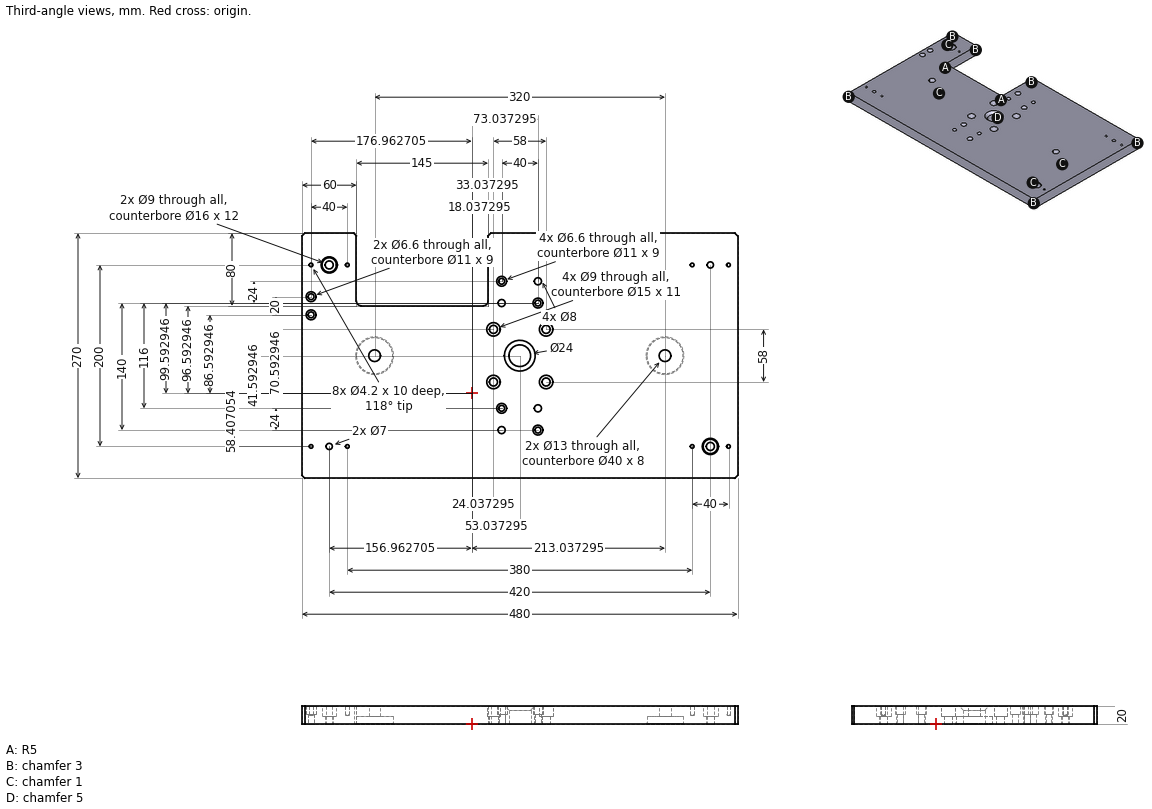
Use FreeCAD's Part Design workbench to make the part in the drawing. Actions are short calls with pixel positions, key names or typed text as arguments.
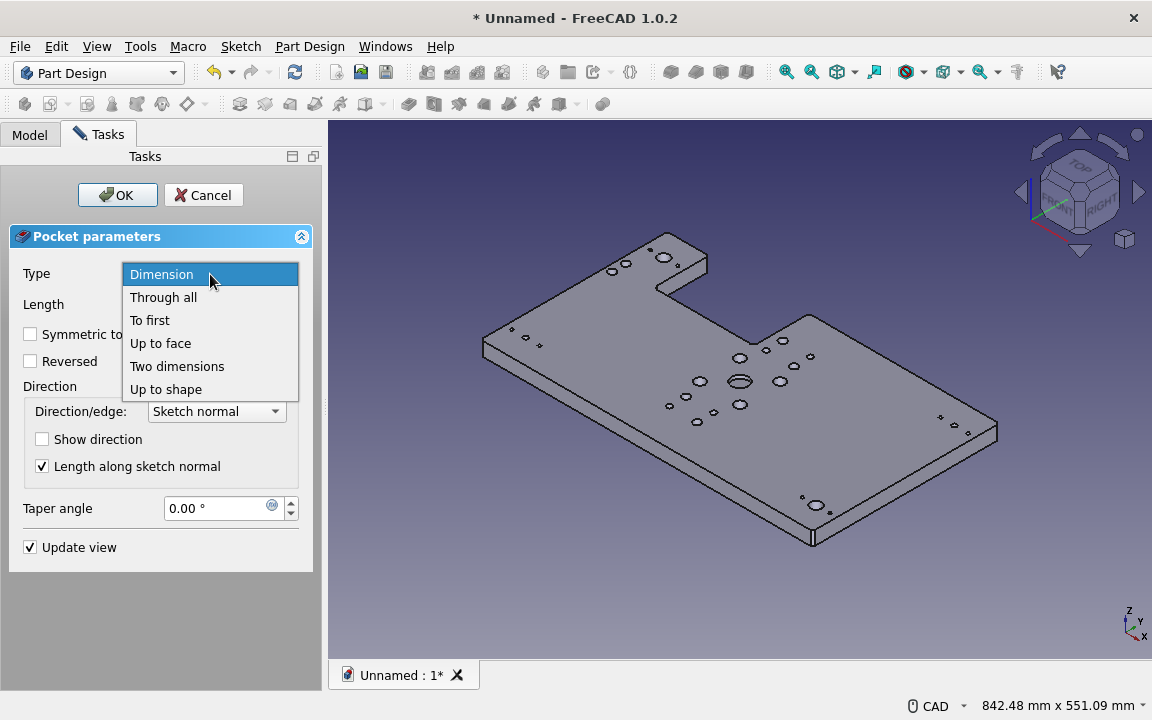
click(208, 298)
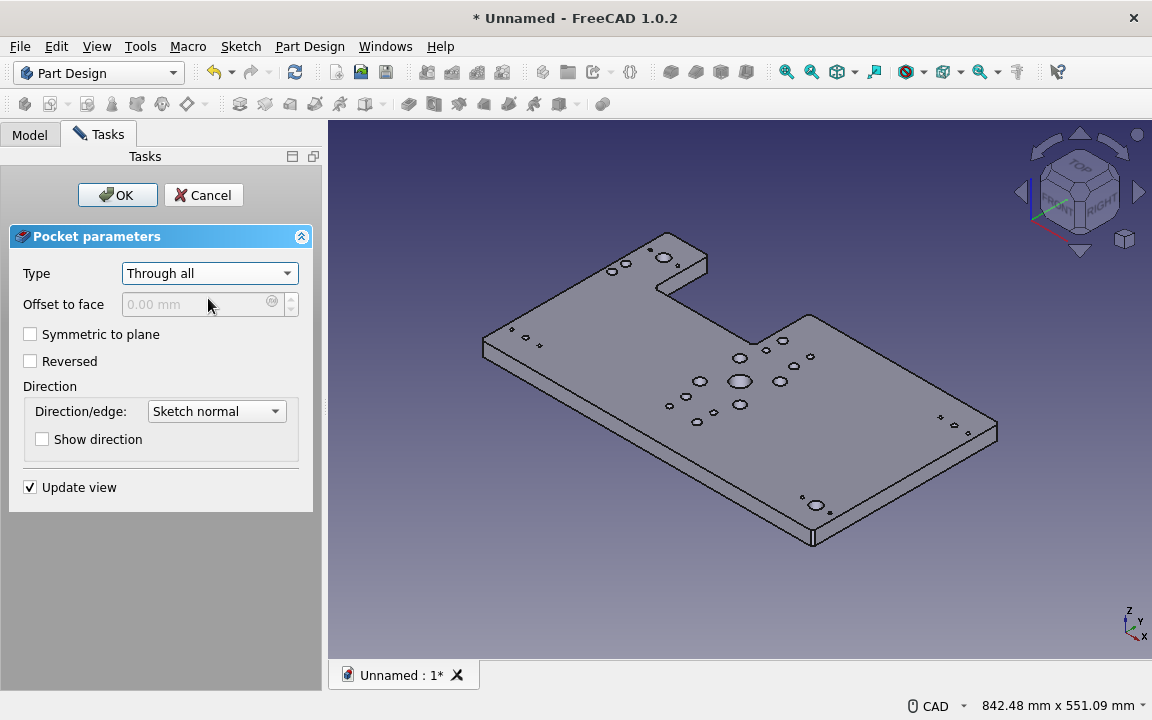
click(118, 195)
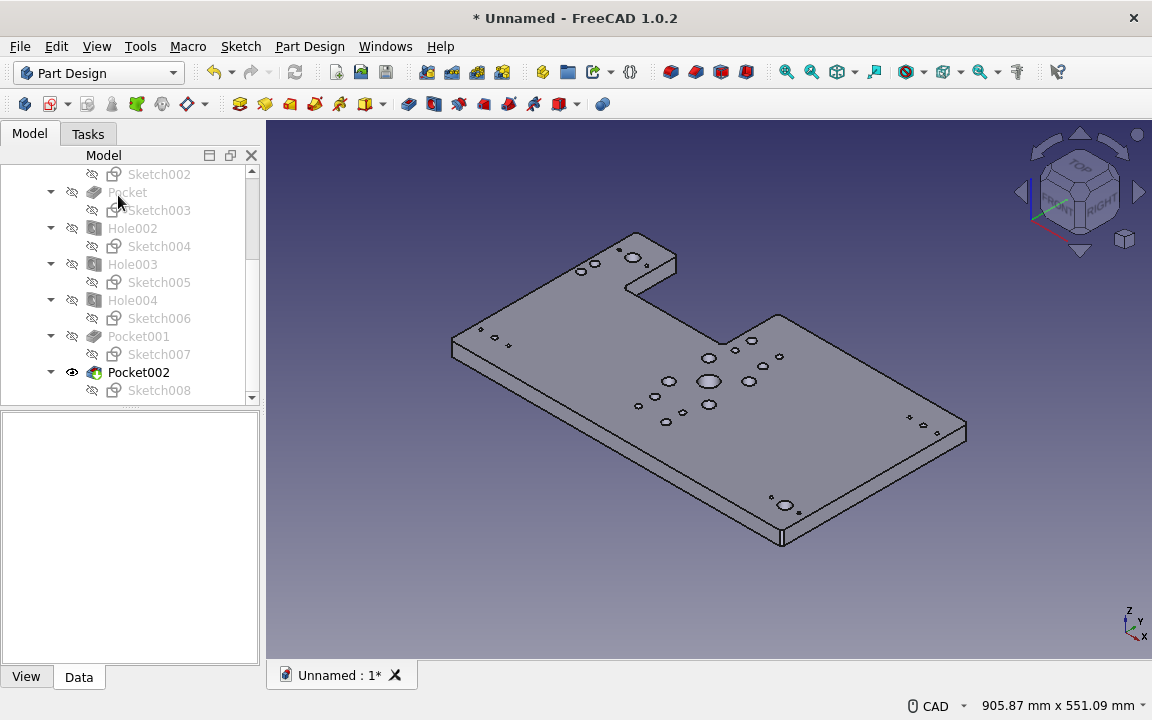
click(50, 104)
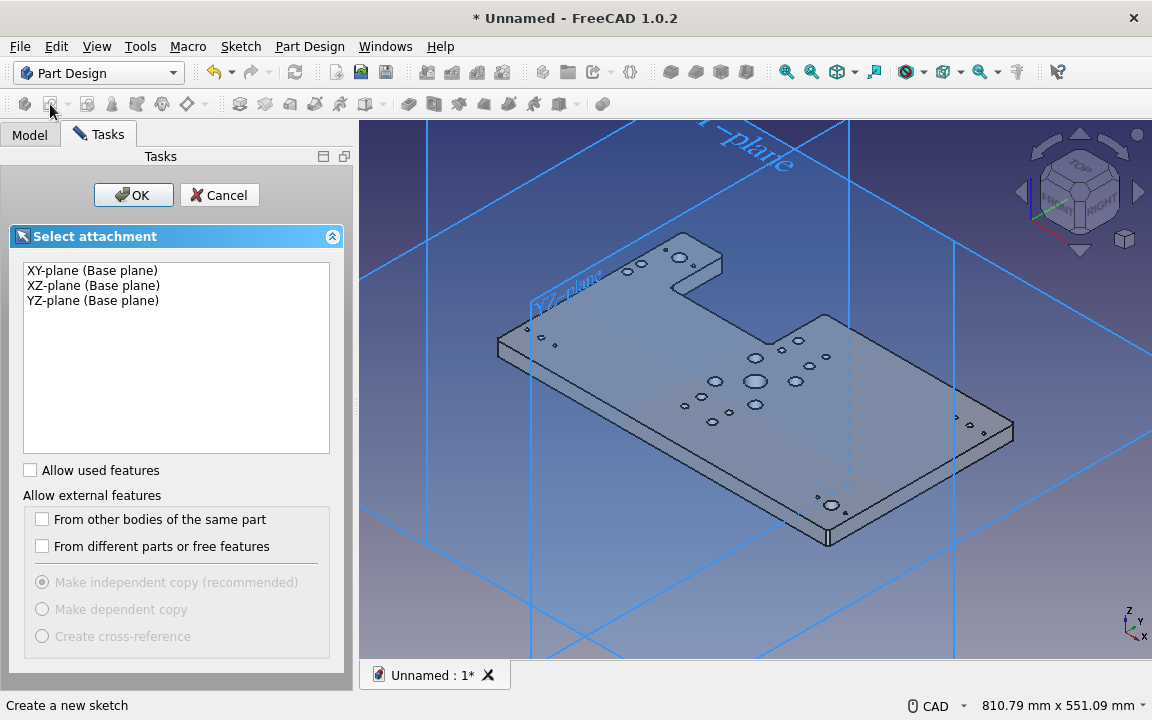
click(84, 270)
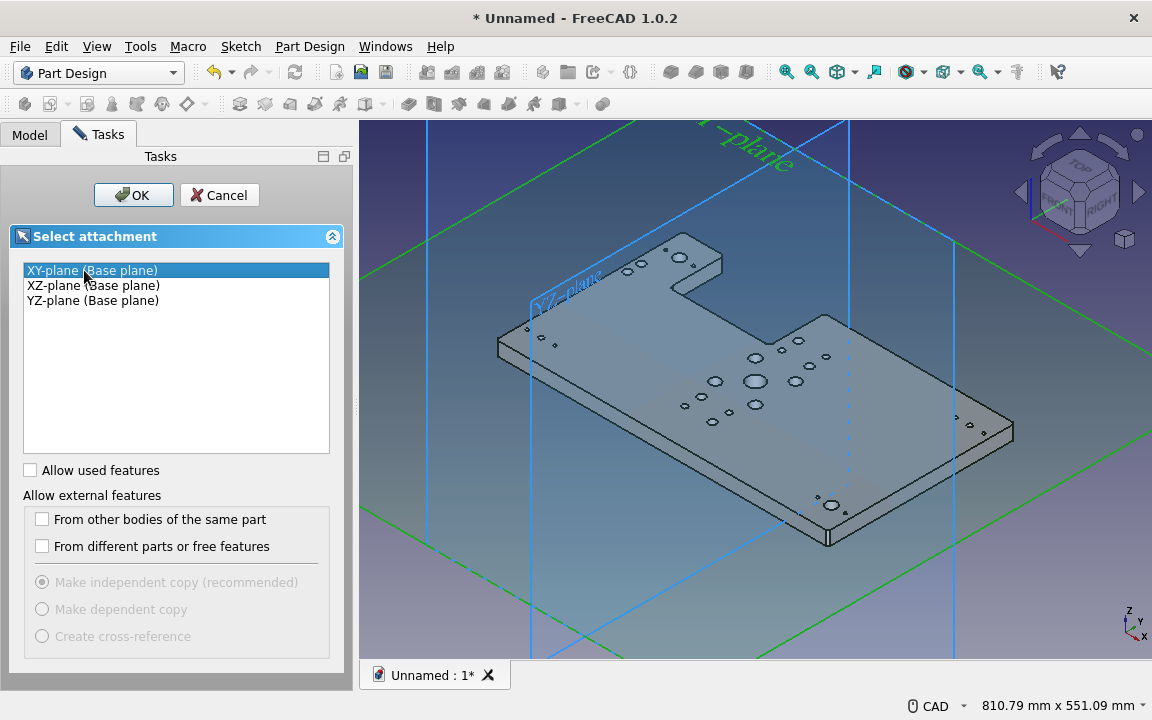
click(134, 195)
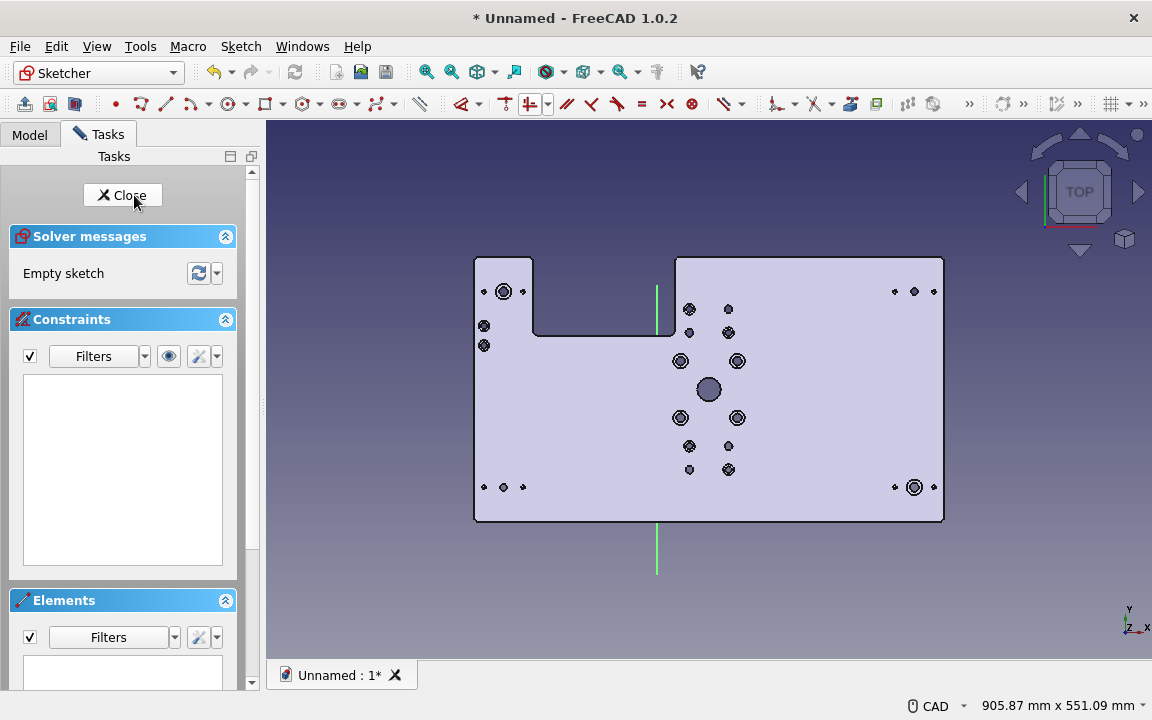
key(q)
key(s)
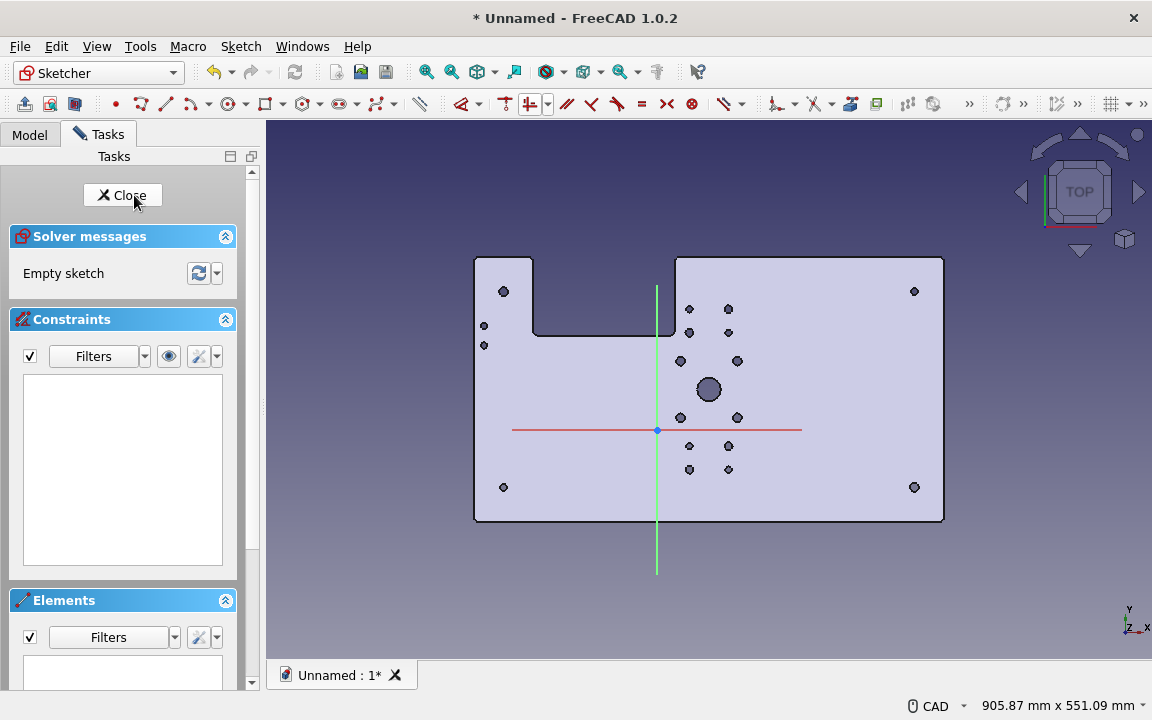
scroll(848, 442, up, 2)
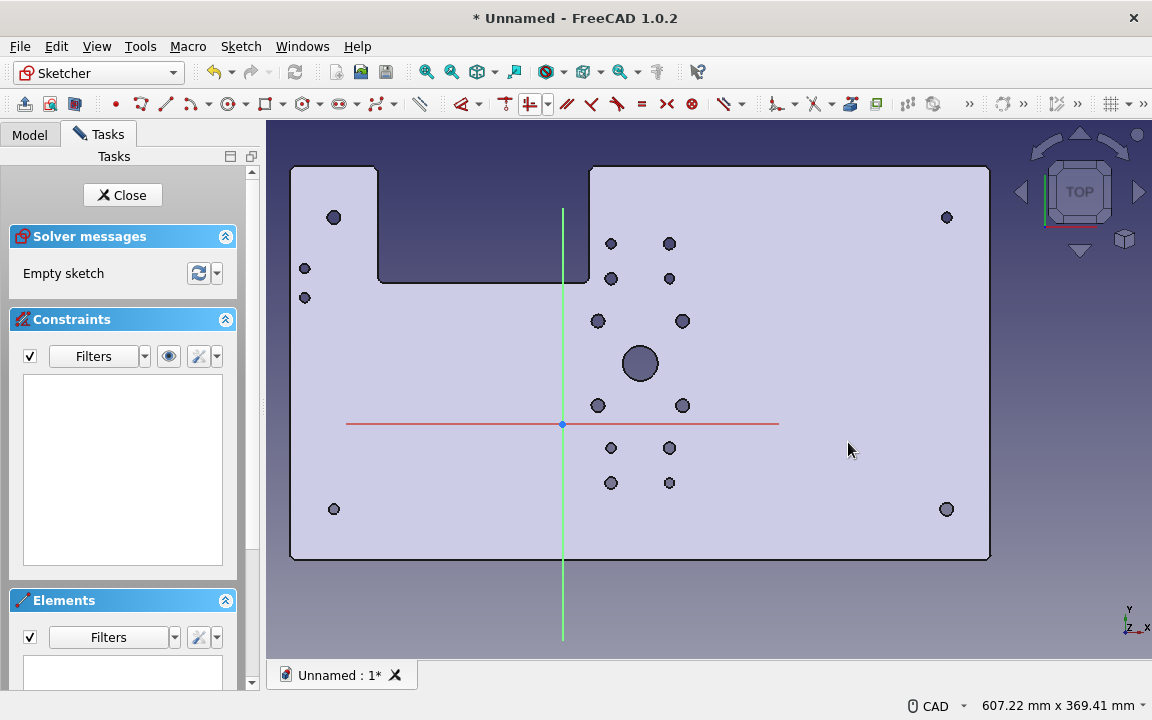
key(g)
key(c)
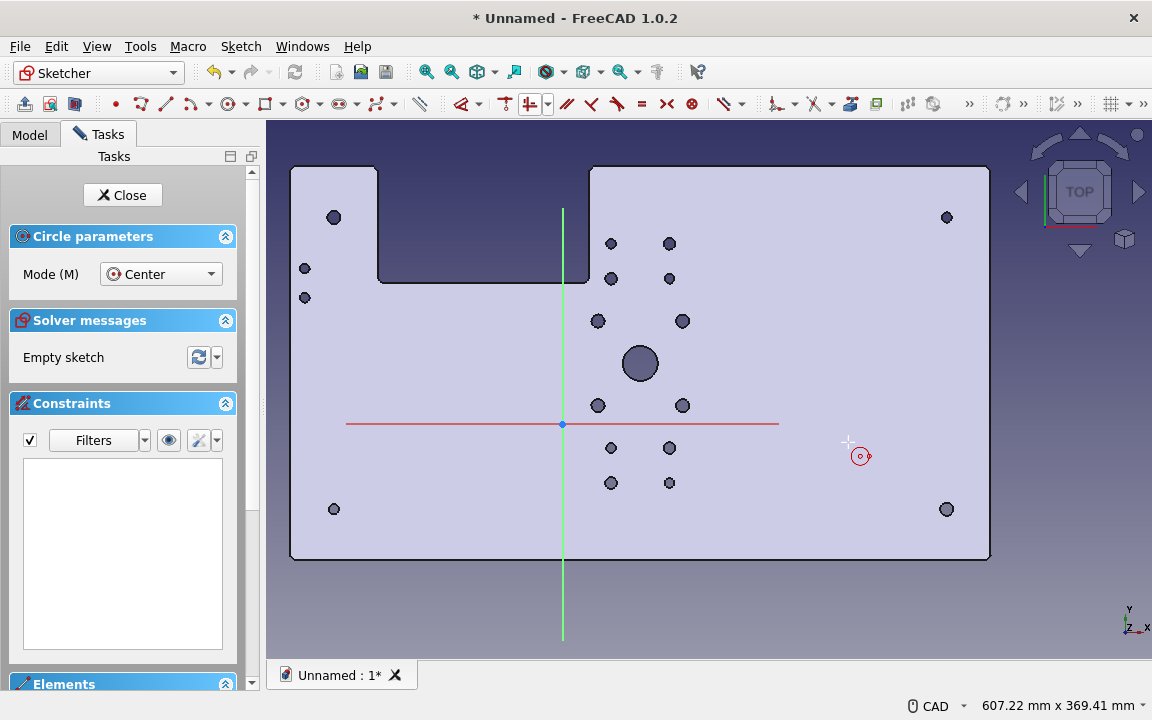
scroll(874, 363, up, 5)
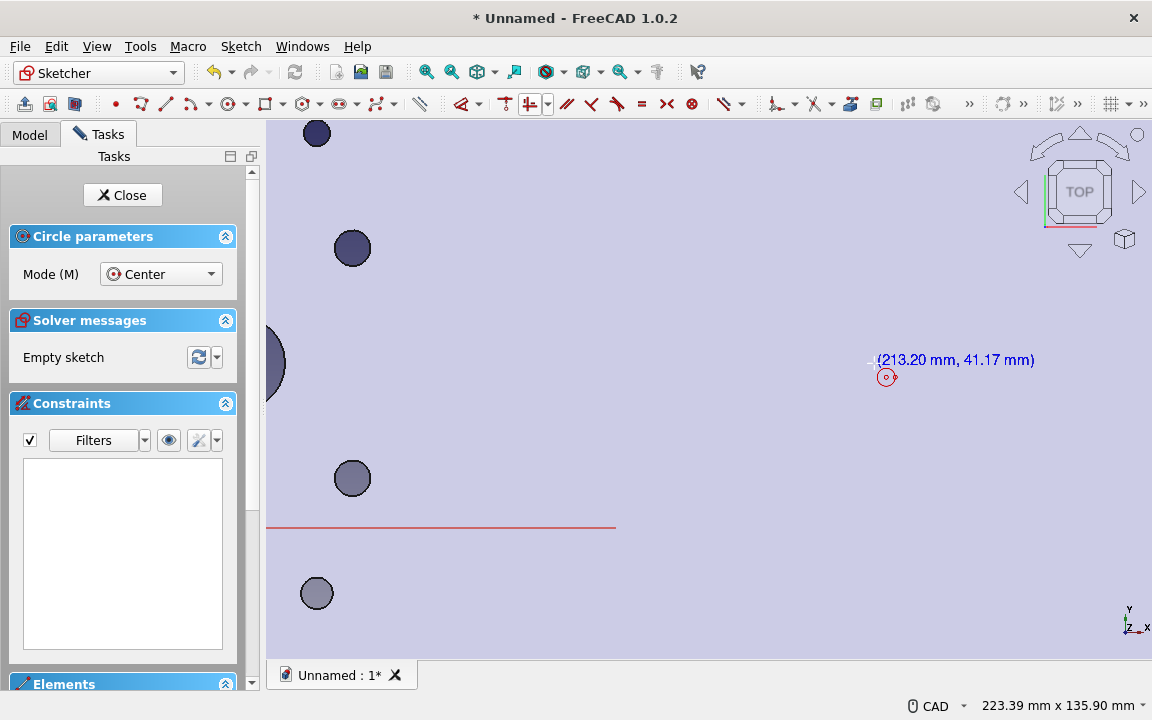
click(872, 363)
click(890, 345)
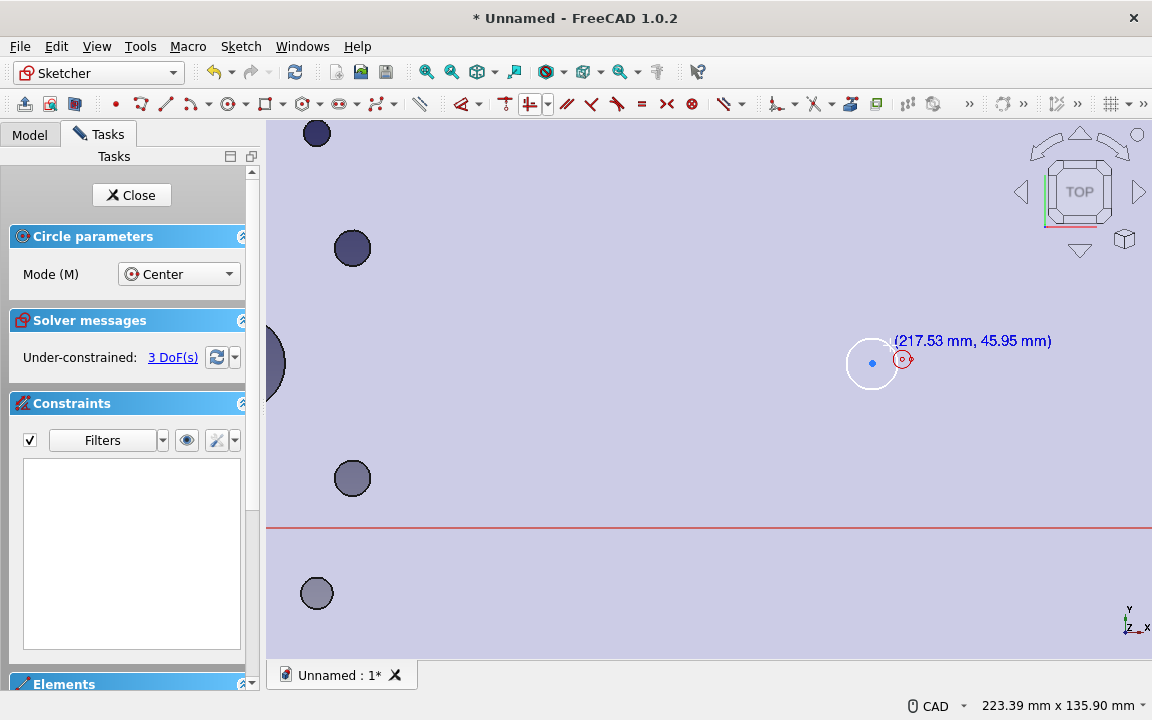
scroll(875, 364, down, 5)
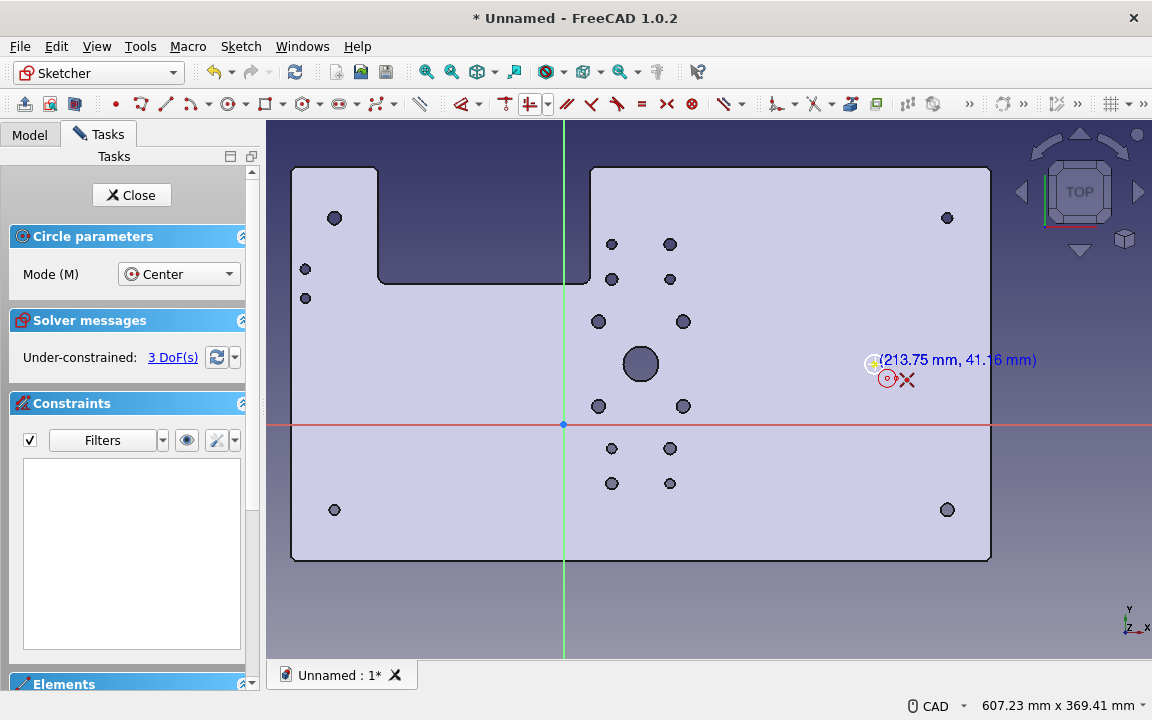
scroll(407, 364, up, 5)